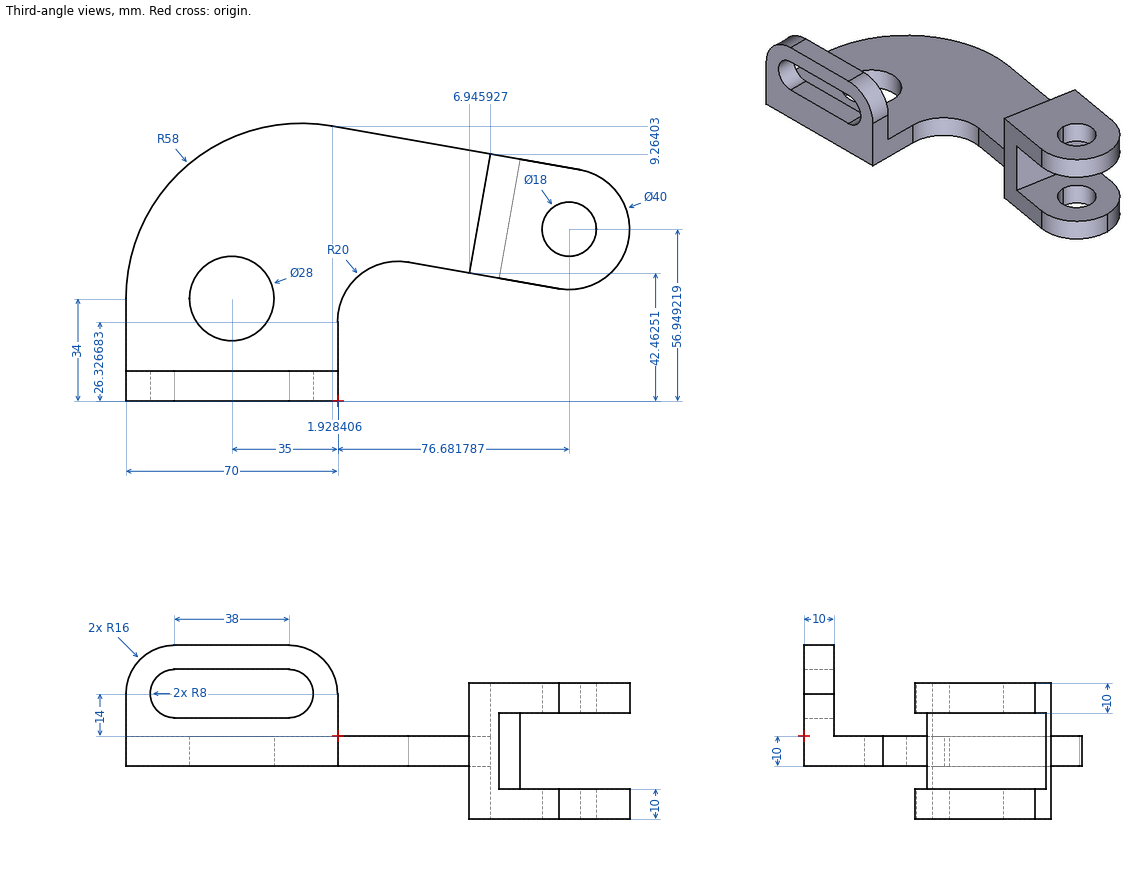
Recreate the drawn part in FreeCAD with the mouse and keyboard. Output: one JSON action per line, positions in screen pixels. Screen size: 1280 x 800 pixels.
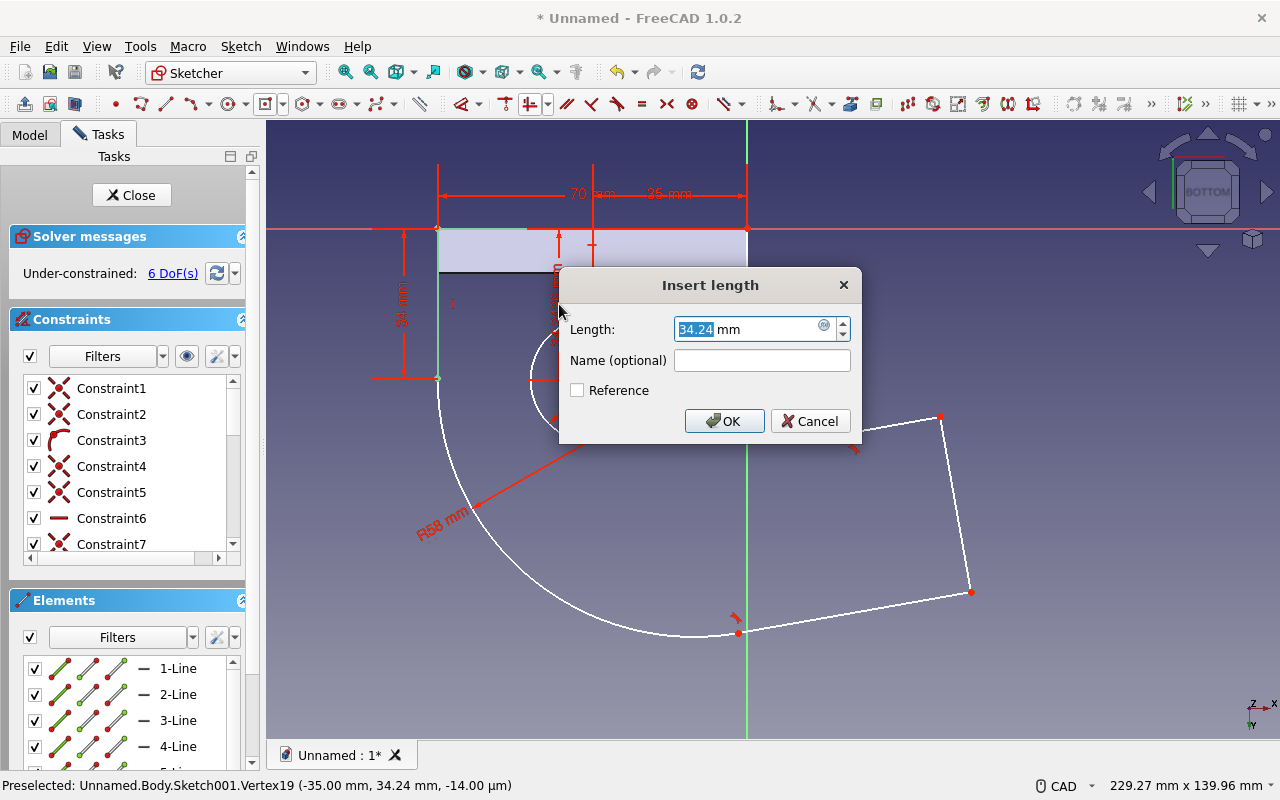
{"action": "type", "text": "34"}
{"action": "key", "text": "Return"}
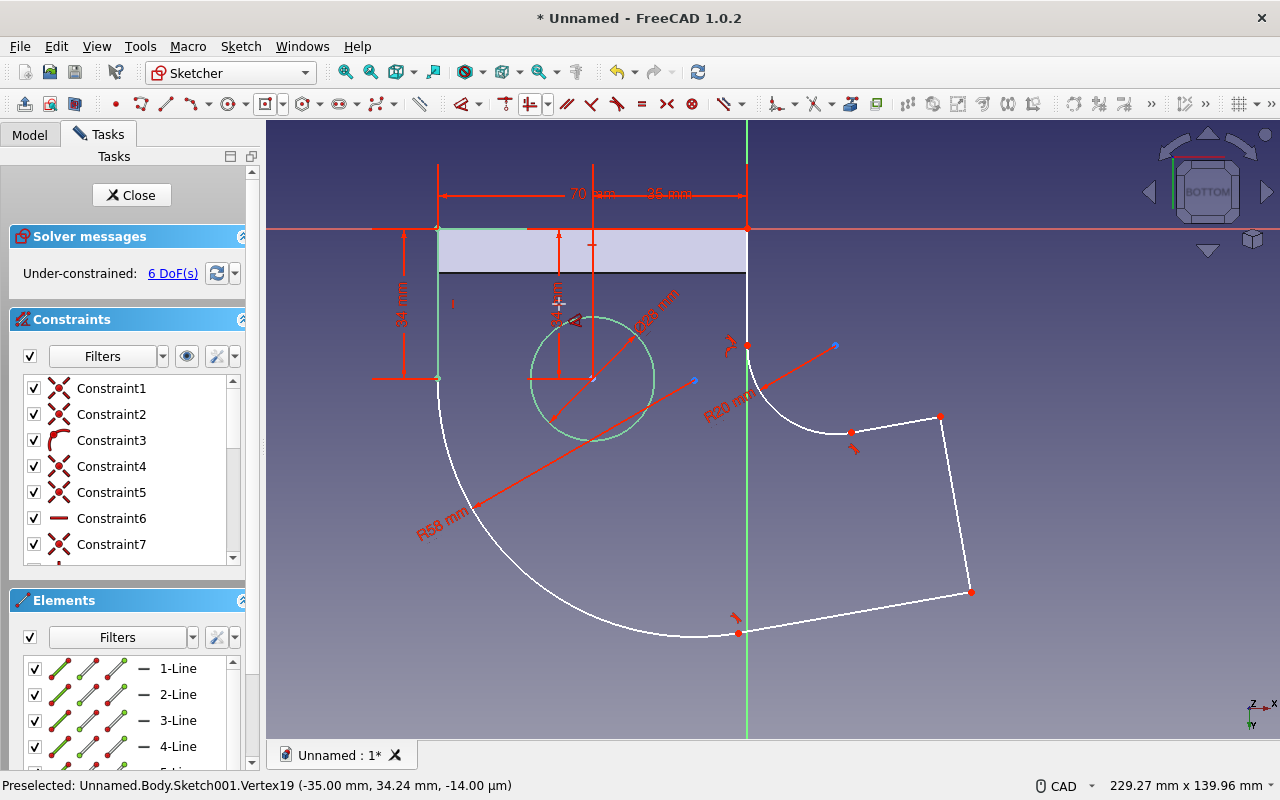
{"action": "left_click", "coordinate": [694, 380]}
{"action": "left_click", "coordinate": [781, 304]}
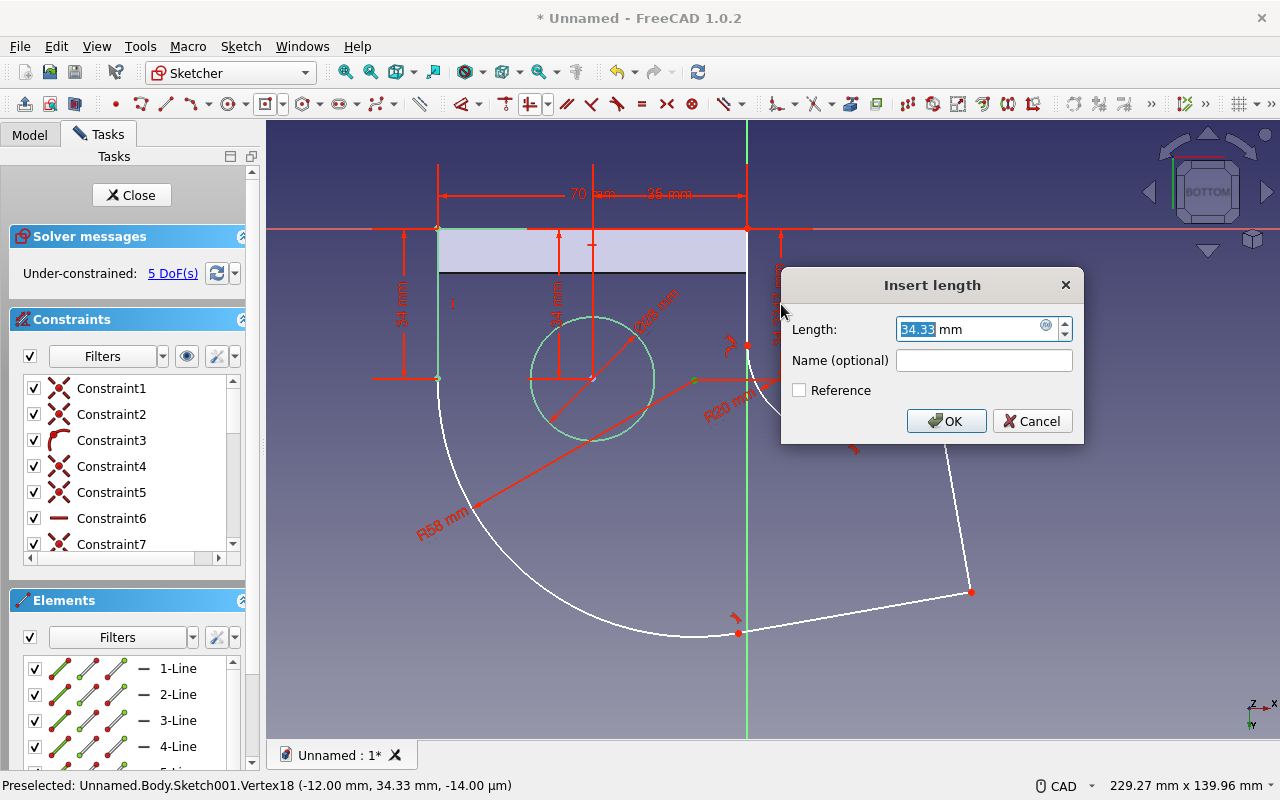
{"action": "type", "text": "34"}
{"action": "key", "text": "Return"}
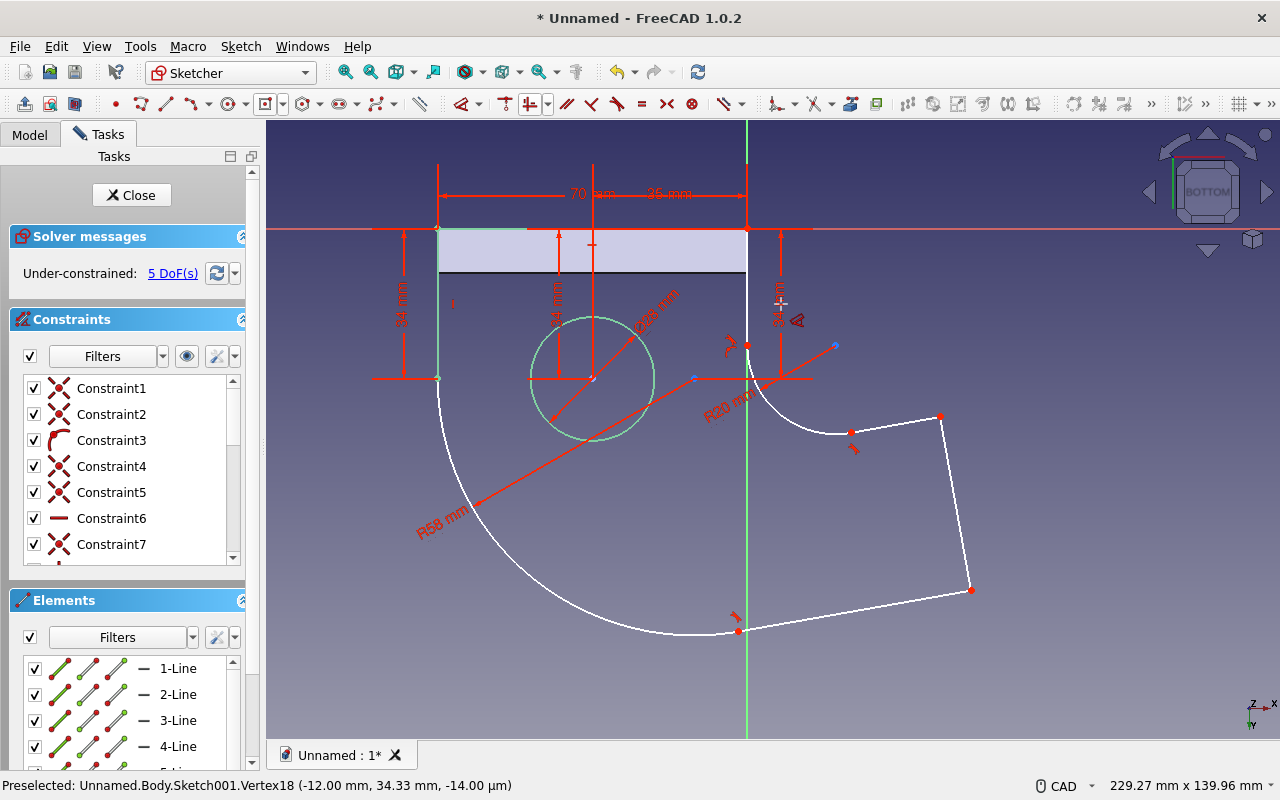
{"action": "left_click", "coordinate": [808, 619]}
{"action": "left_click", "coordinate": [1005, 611]}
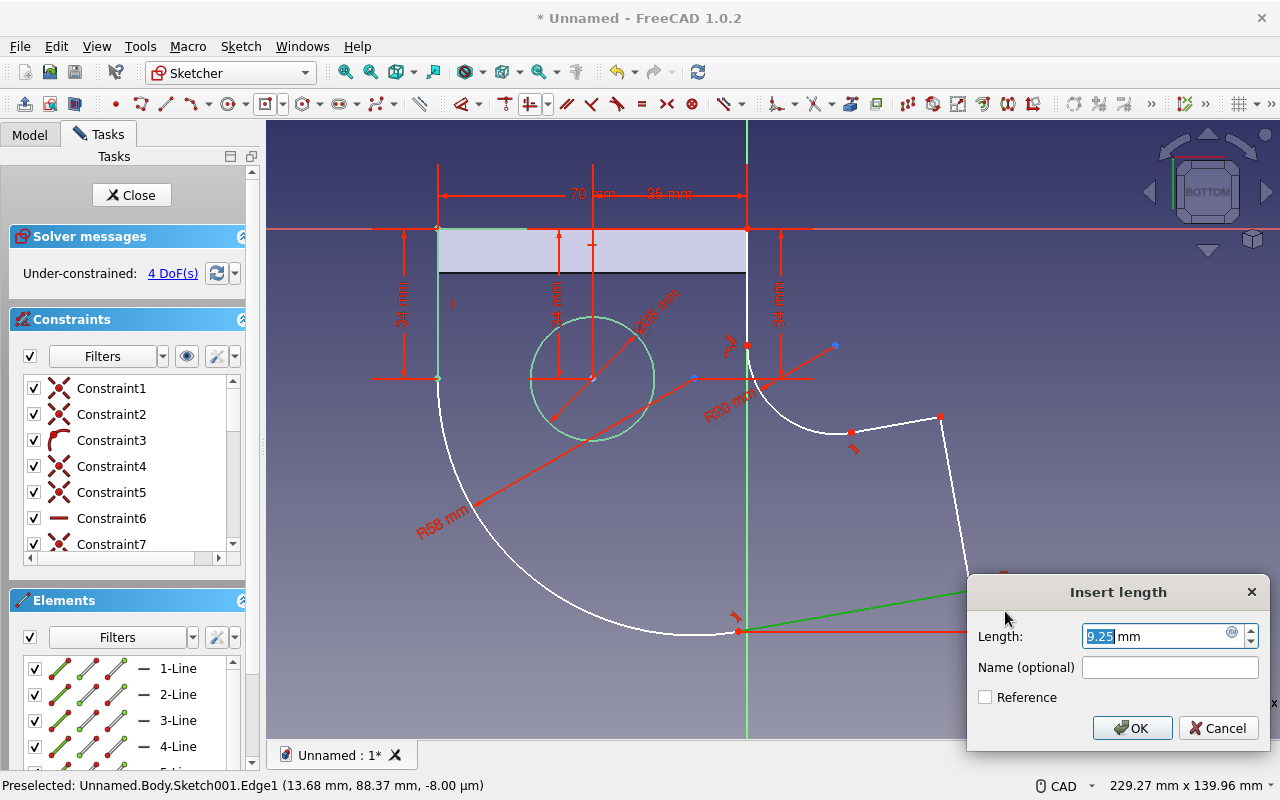
{"action": "type", "text": "9.26403"}
{"action": "key", "text": "Return"}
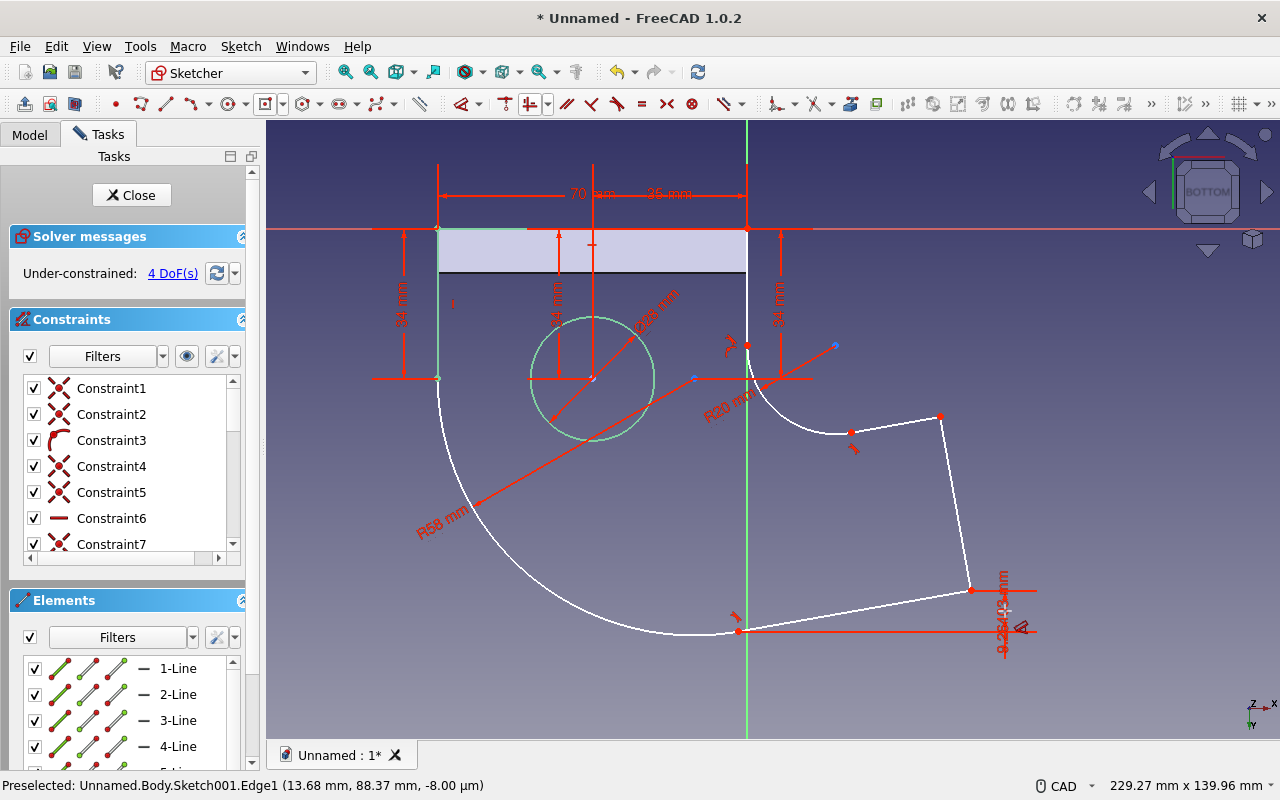
{"action": "left_click", "coordinate": [747, 311]}
{"action": "left_click", "coordinate": [781, 260]}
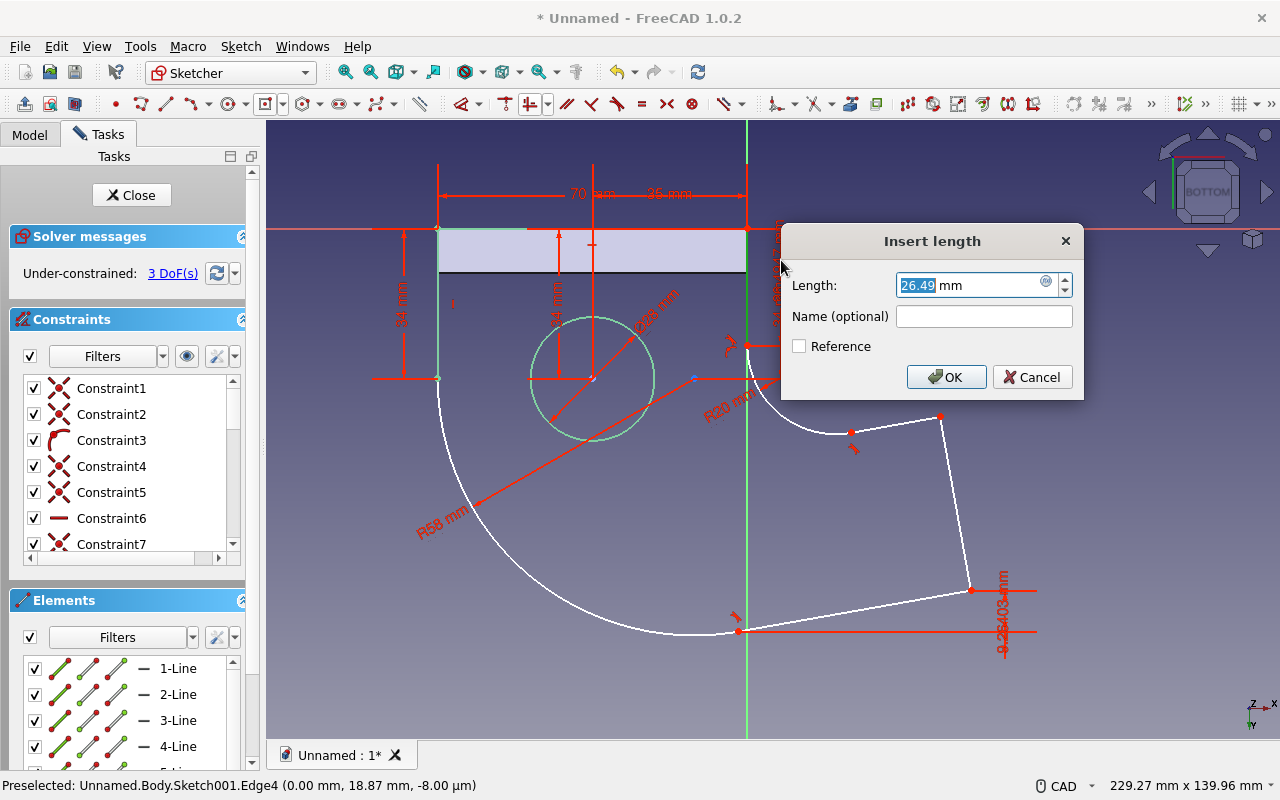
{"action": "type", "text": "26.326683"}
{"action": "key", "text": "Return"}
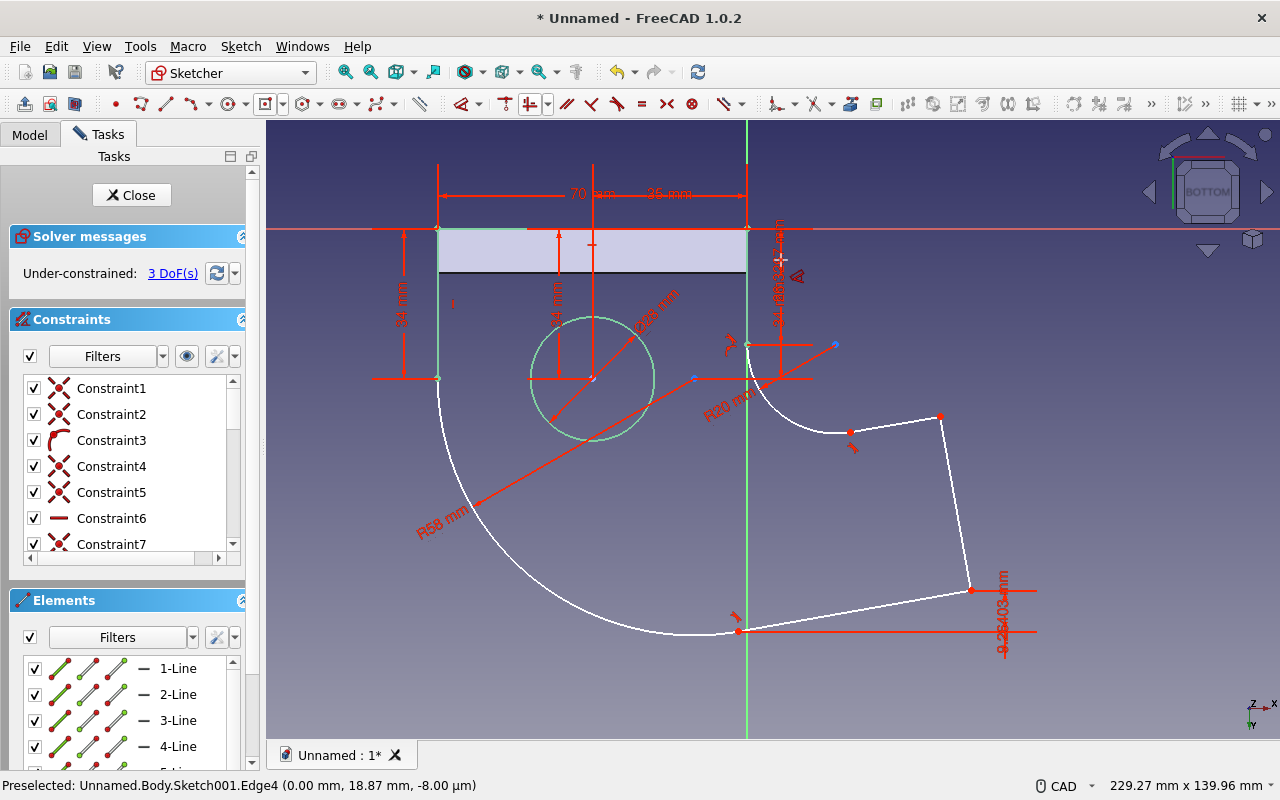
{"action": "scroll", "coordinate": [739, 632], "scroll_direction": "up", "scroll_amount": 8}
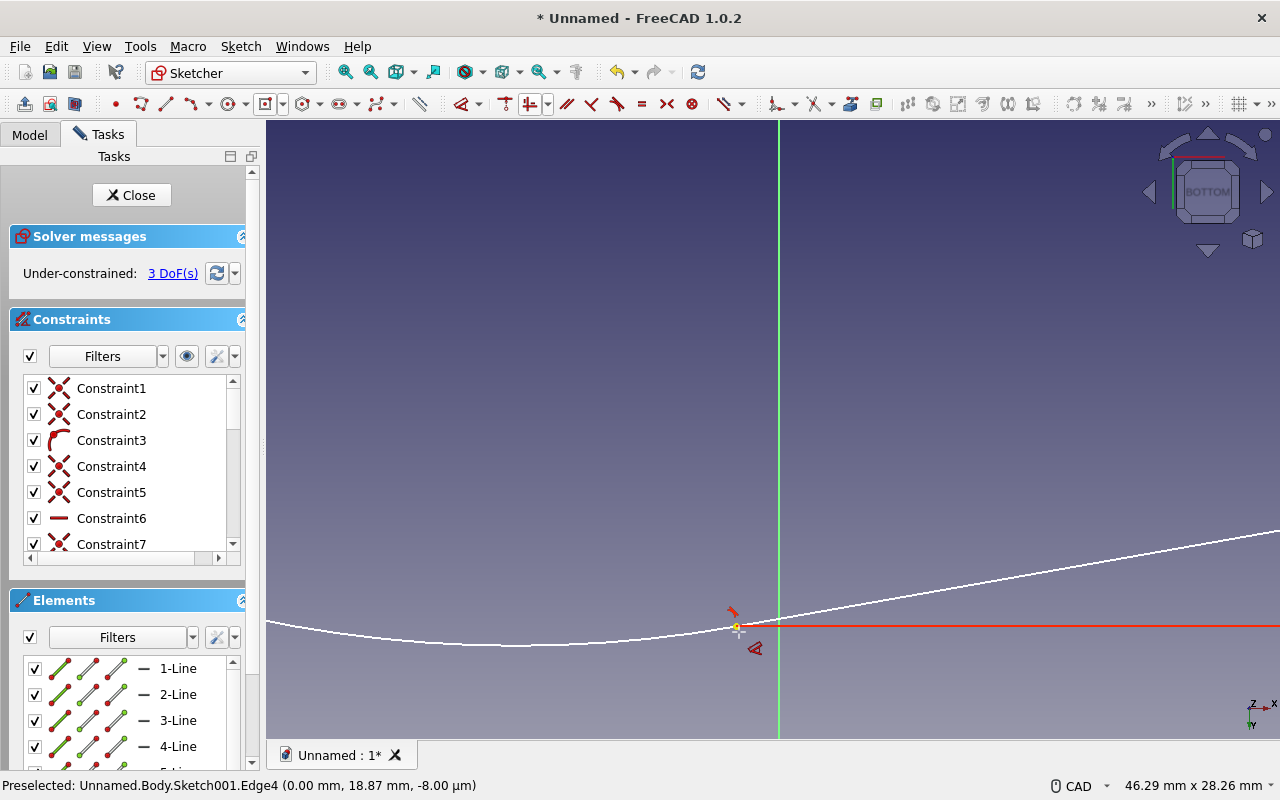
{"action": "left_click", "coordinate": [737, 626]}
{"action": "left_click", "coordinate": [758, 660]}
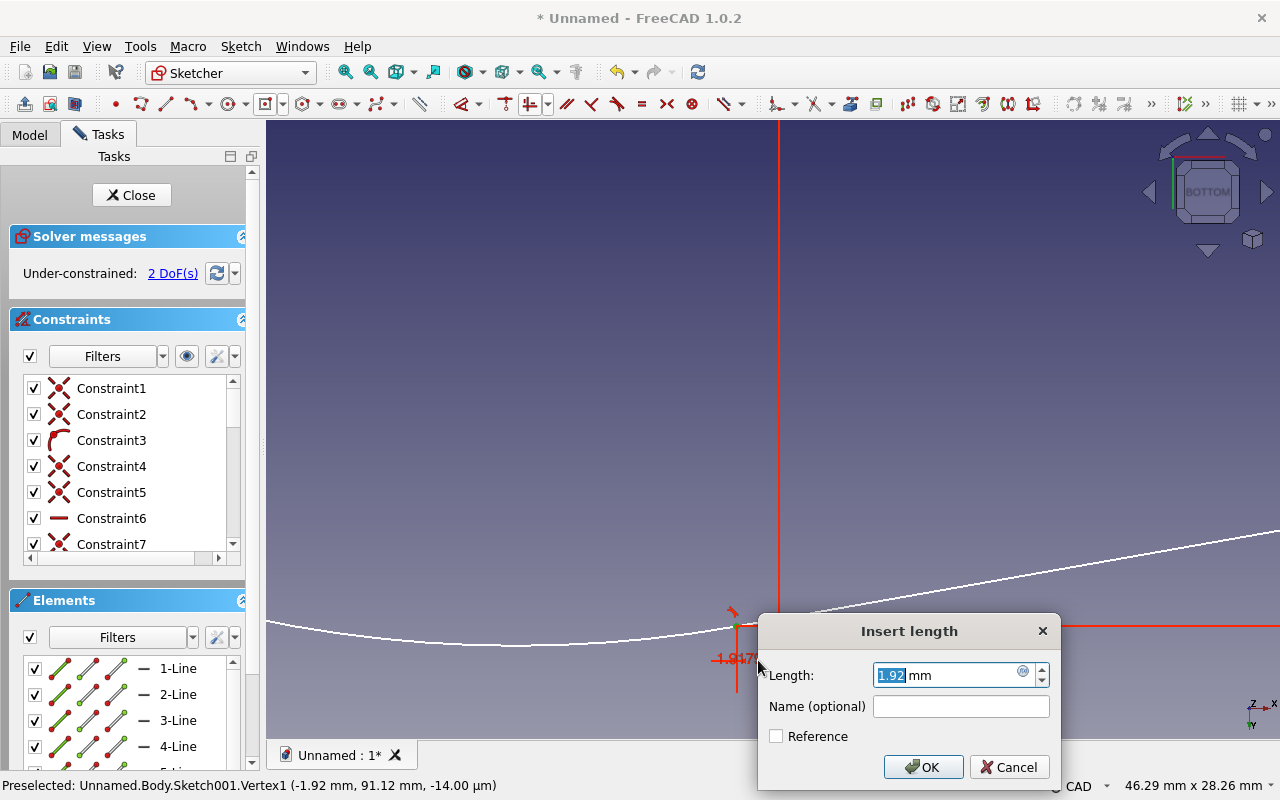
{"action": "type", "text": "1.928406"}
{"action": "key", "text": "Return"}